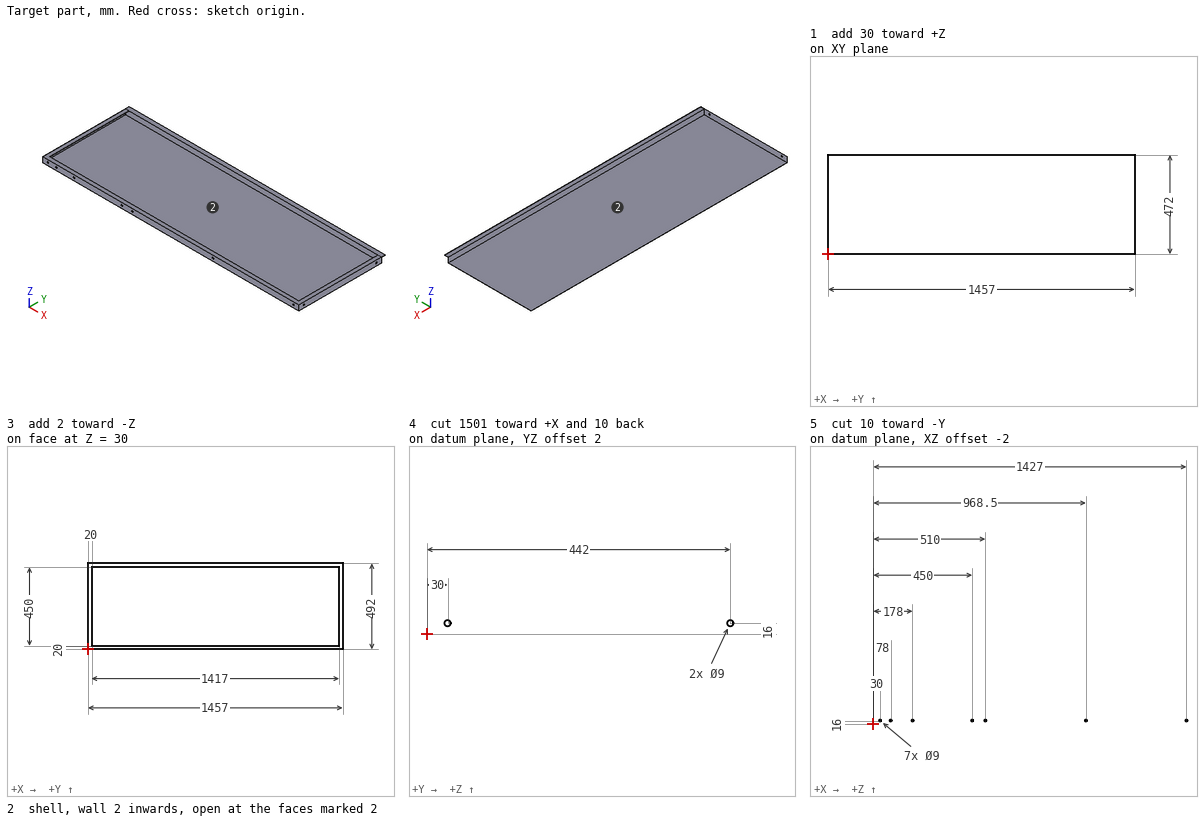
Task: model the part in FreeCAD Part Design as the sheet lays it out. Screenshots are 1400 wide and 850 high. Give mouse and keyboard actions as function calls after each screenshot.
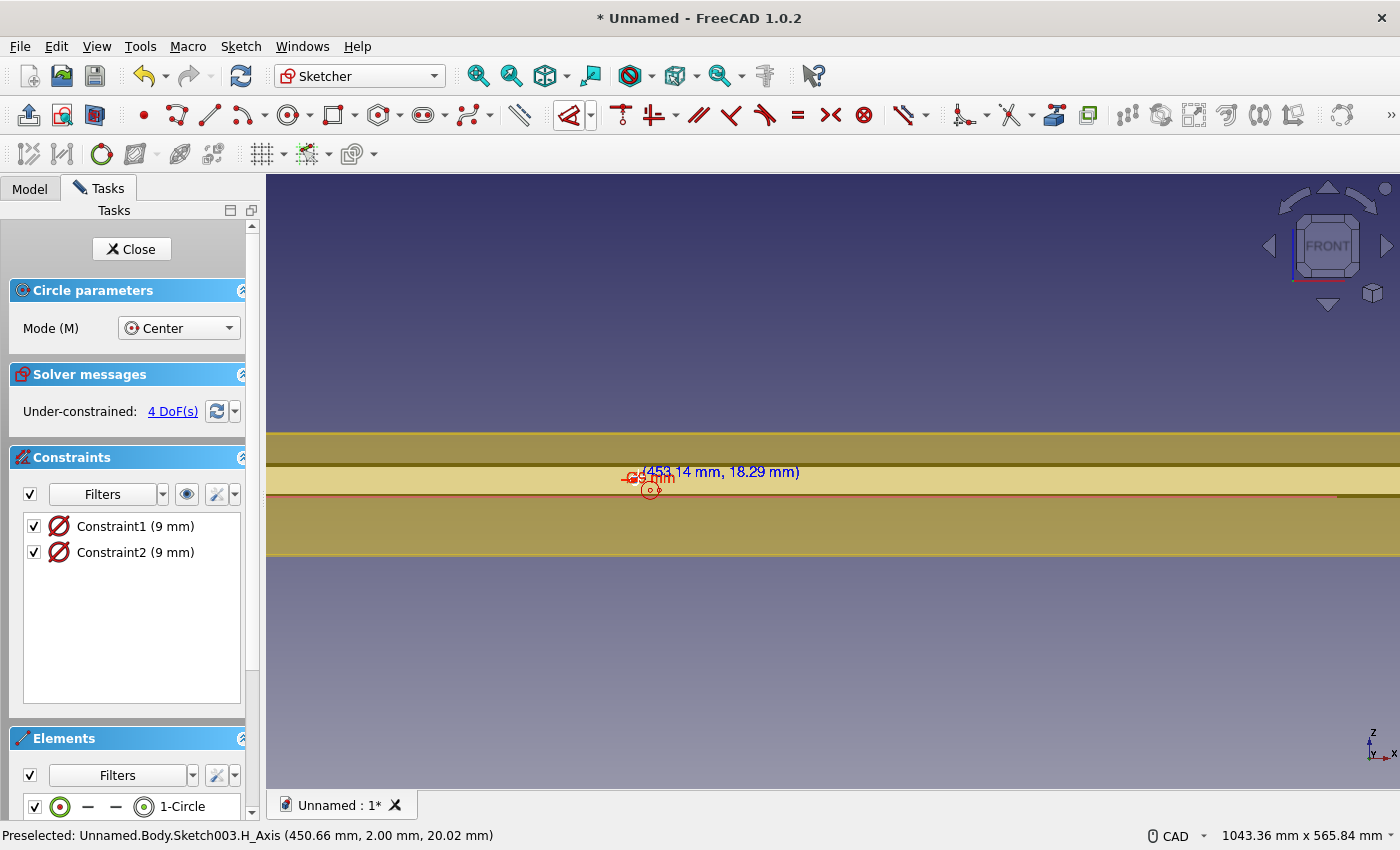
scroll(635, 478, down, 4)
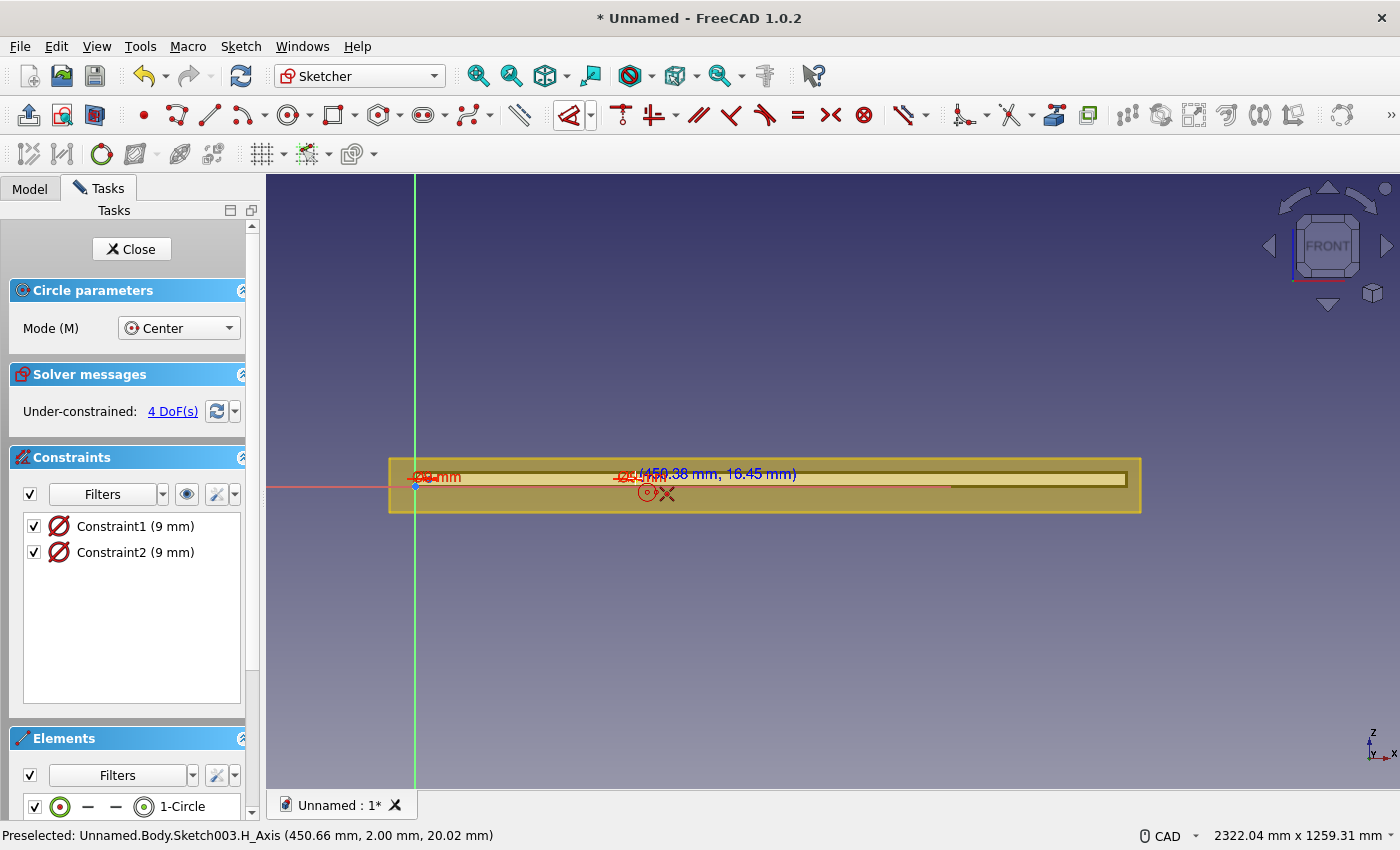
scroll(1112, 479, up, 12)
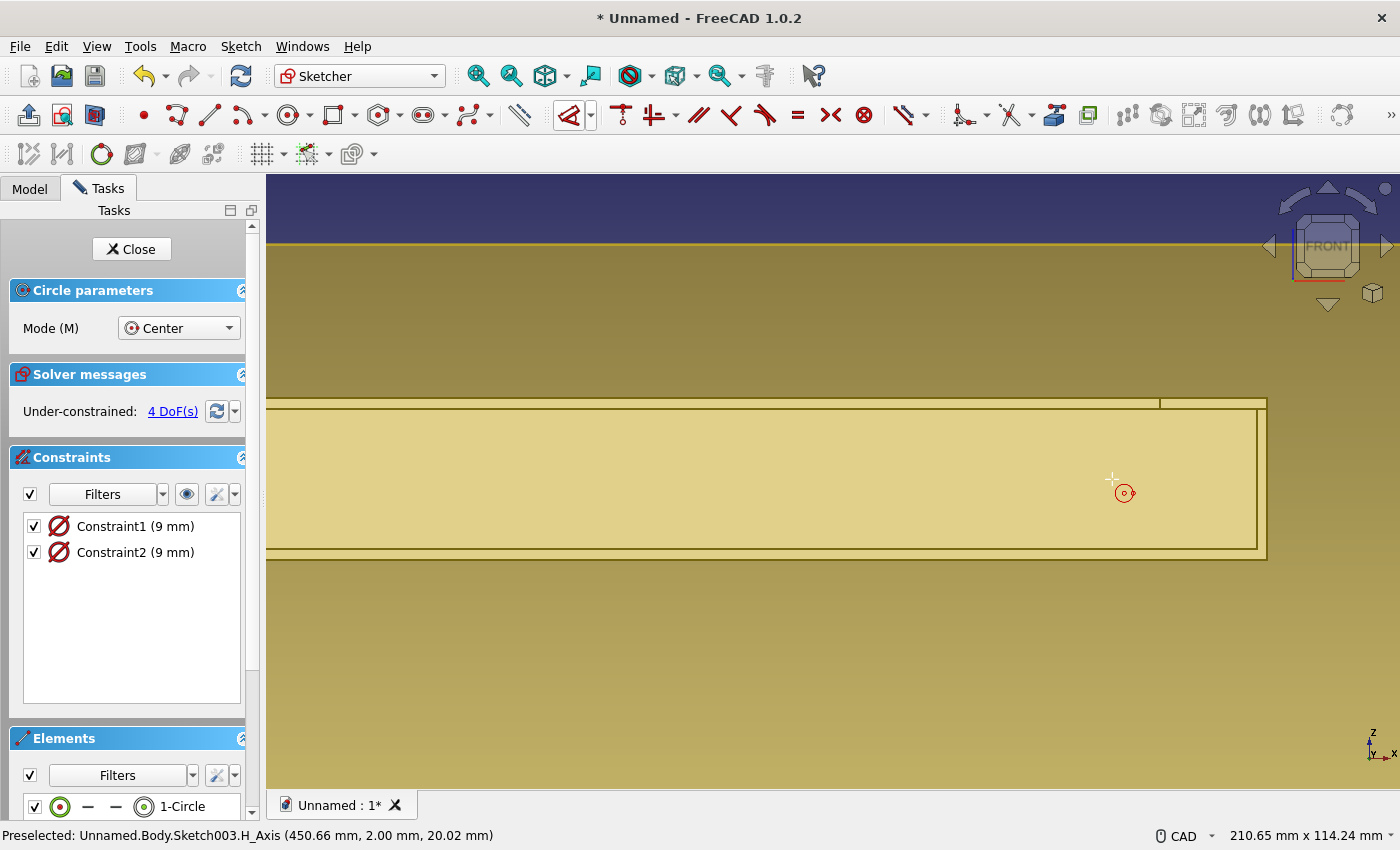
scroll(1112, 479, down, 12)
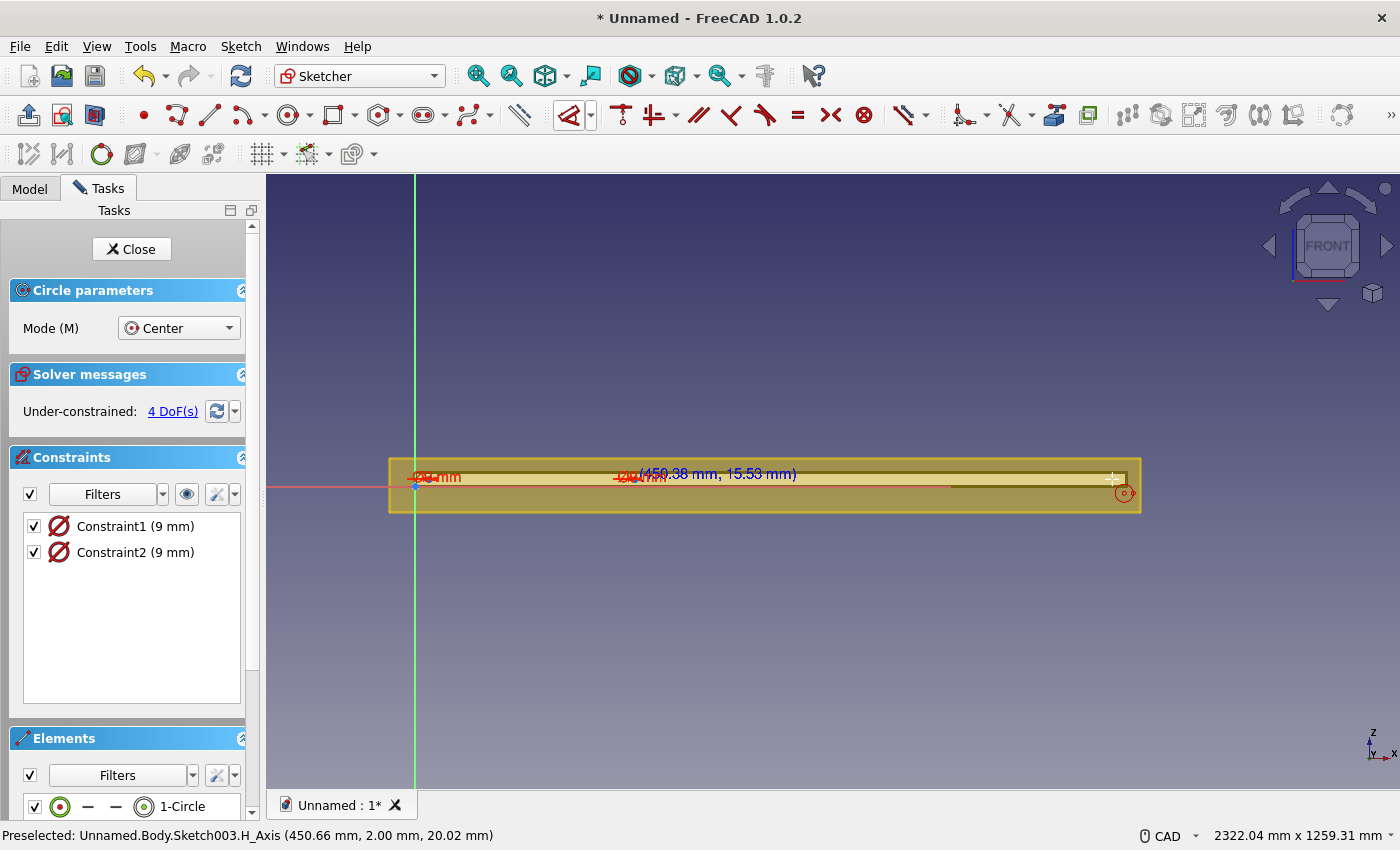
scroll(1112, 479, up, 4)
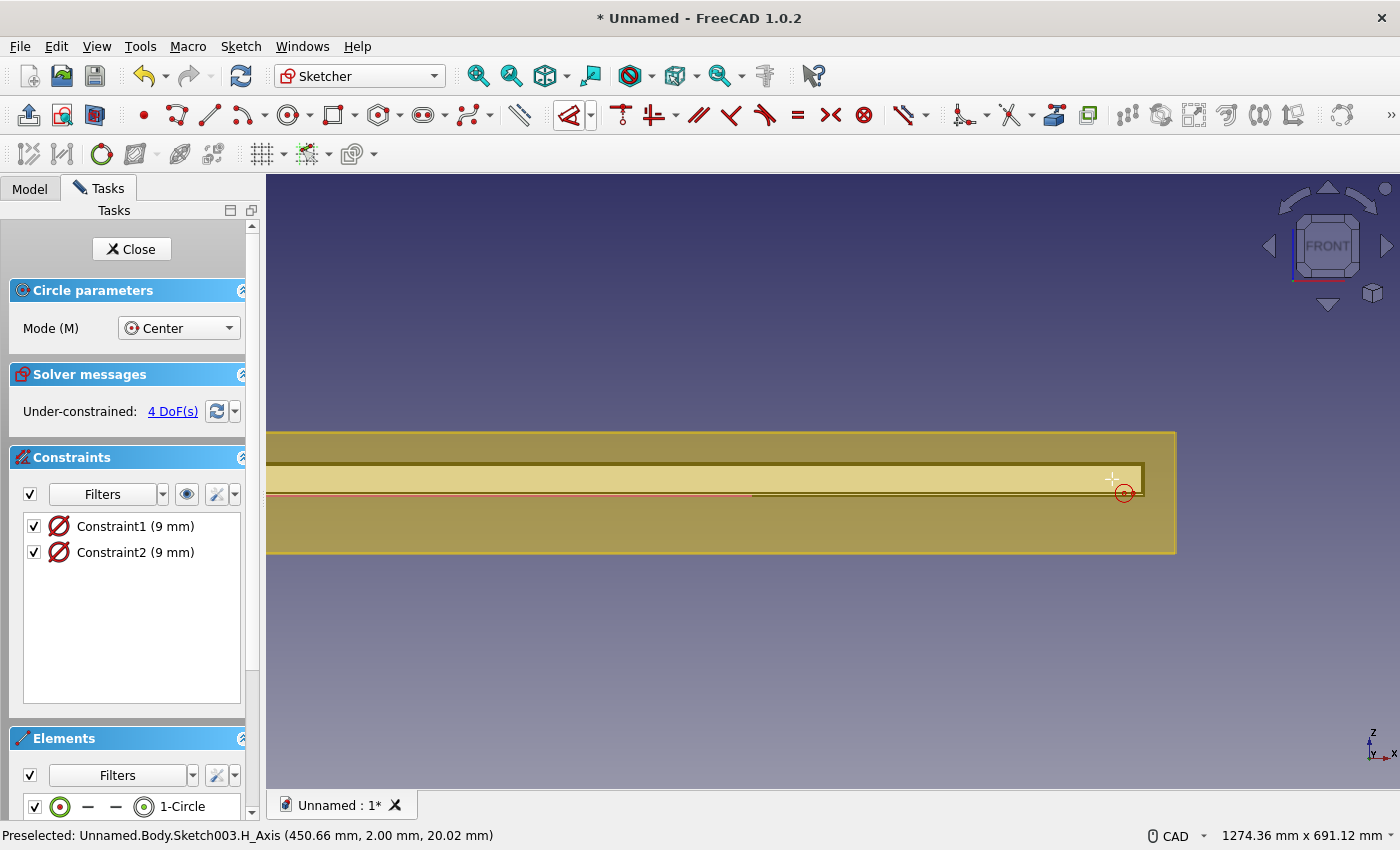
click(1111, 478)
move(1115, 475)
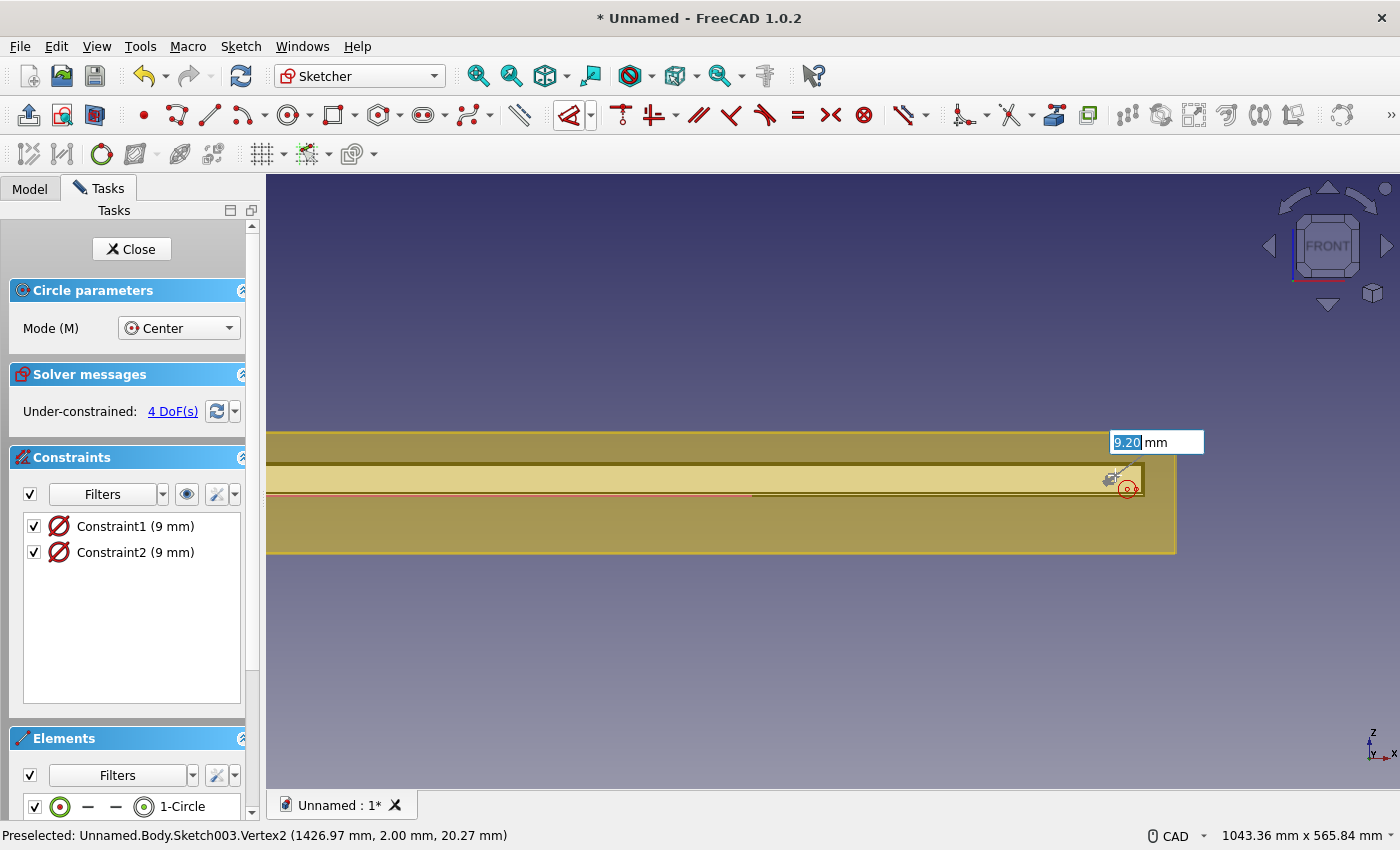
text(9)
key(Return)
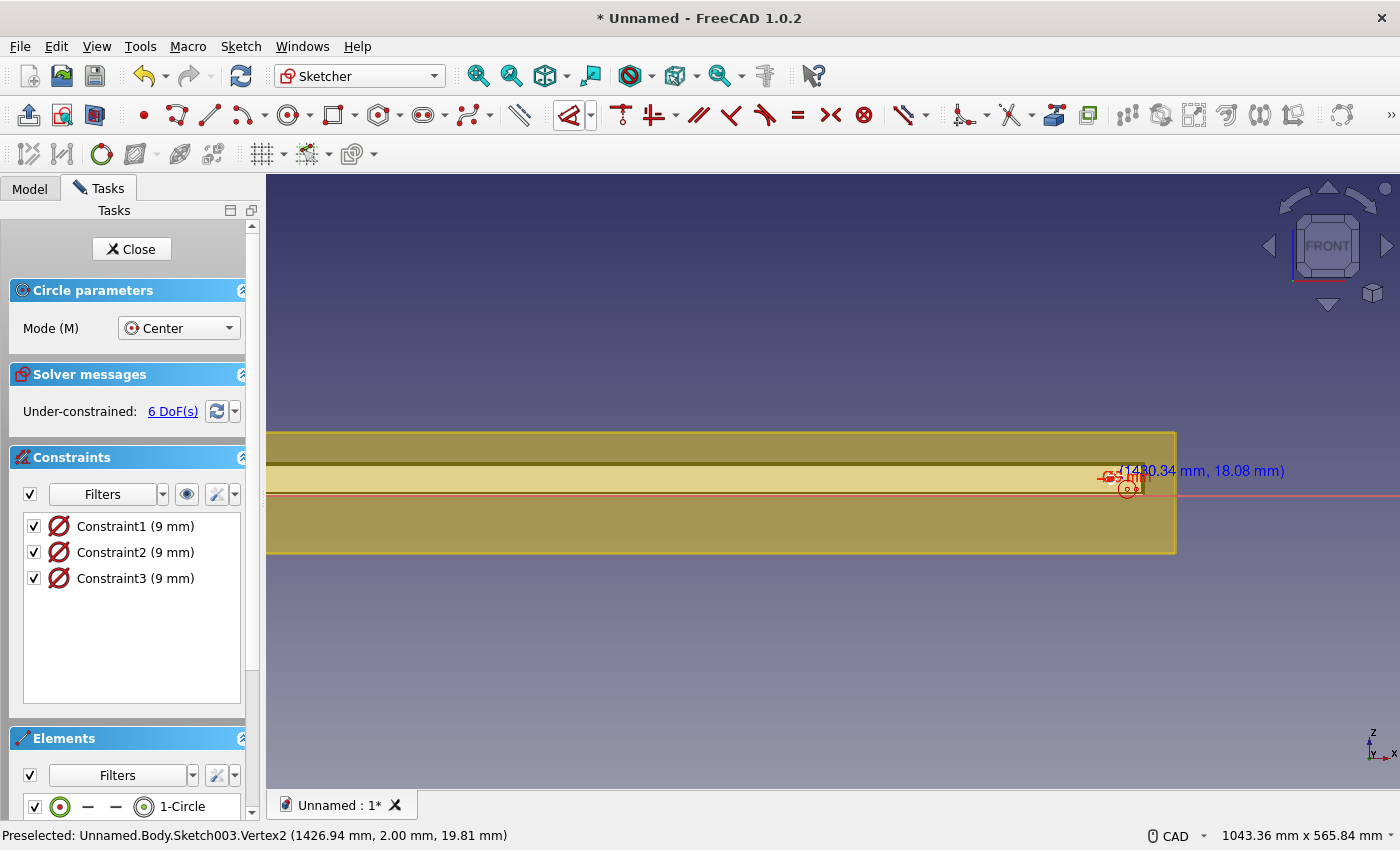
scroll(613, 478, up, 8)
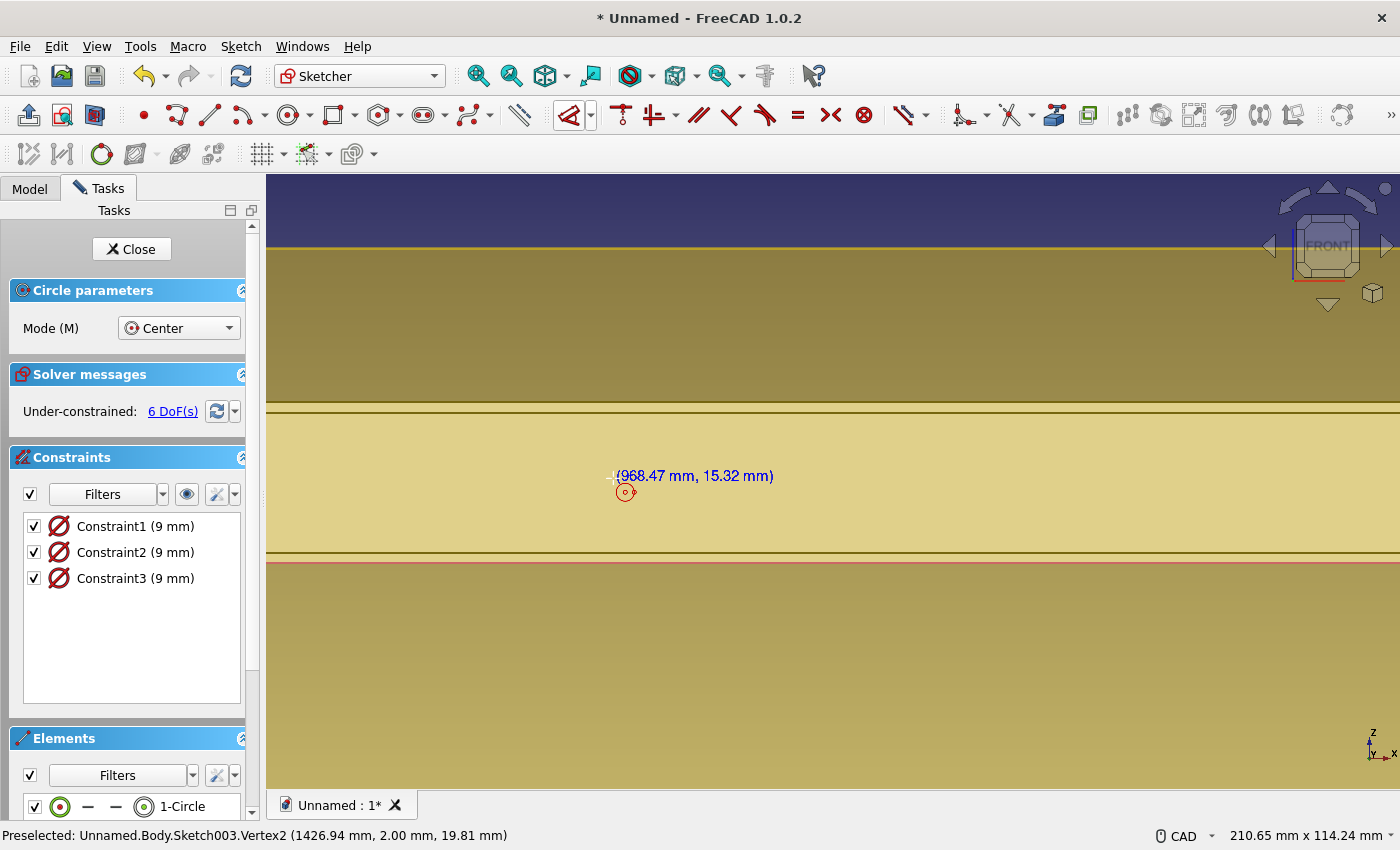
scroll(915, 479, down, 12)